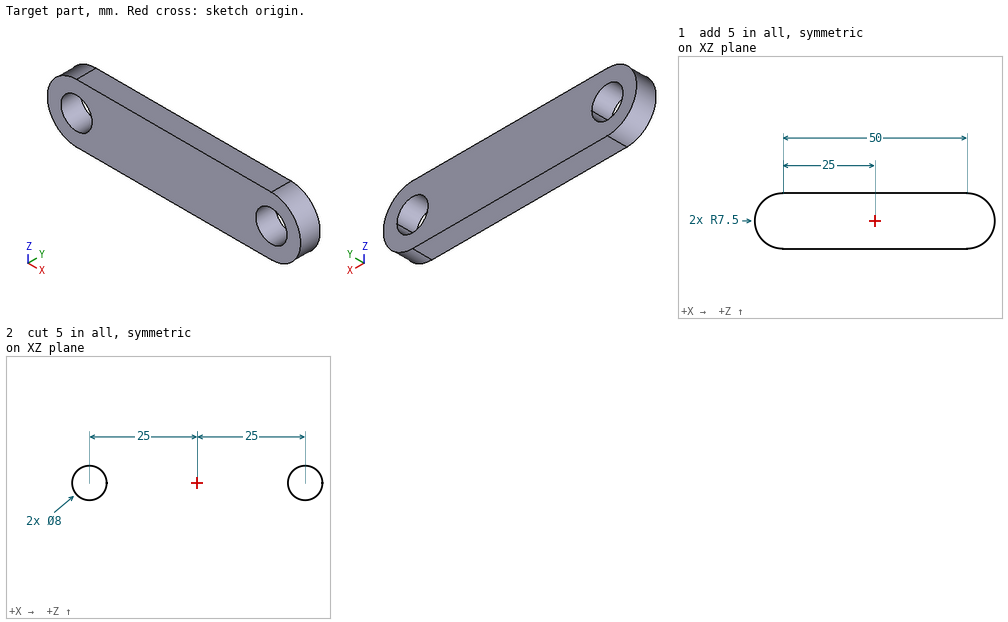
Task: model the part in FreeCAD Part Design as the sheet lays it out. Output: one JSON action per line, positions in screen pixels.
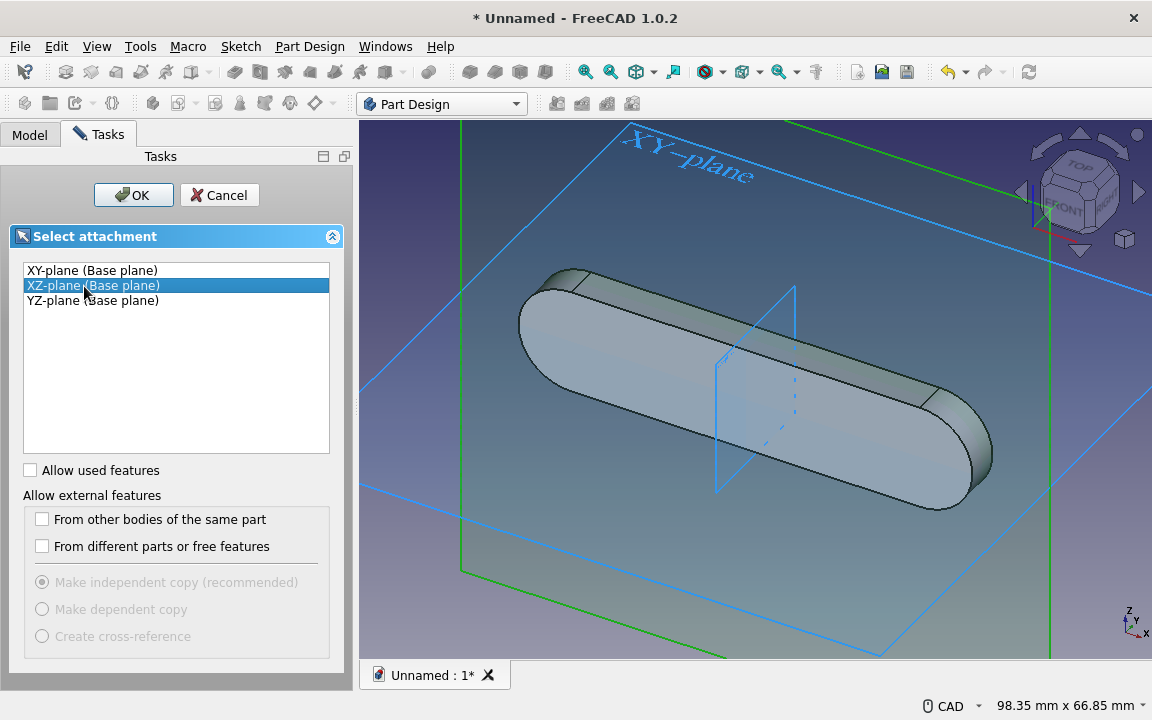
{"action": "left_click", "coordinate": [134, 195]}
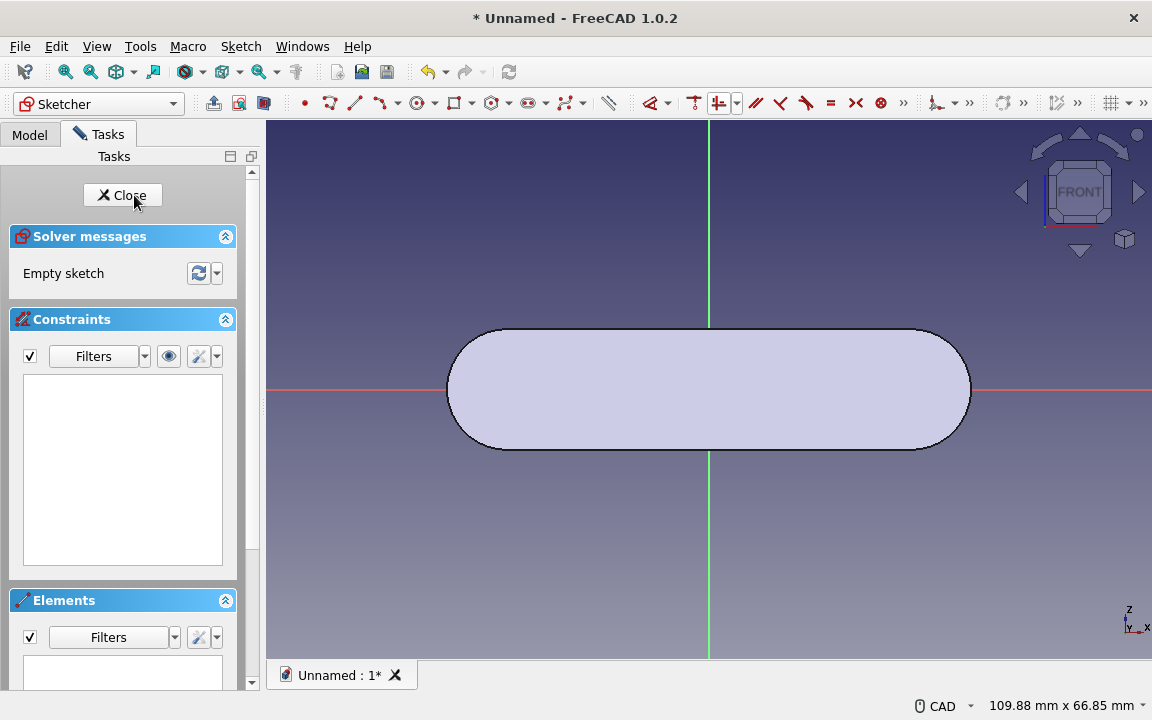
{"action": "left_click", "coordinate": [264, 104]}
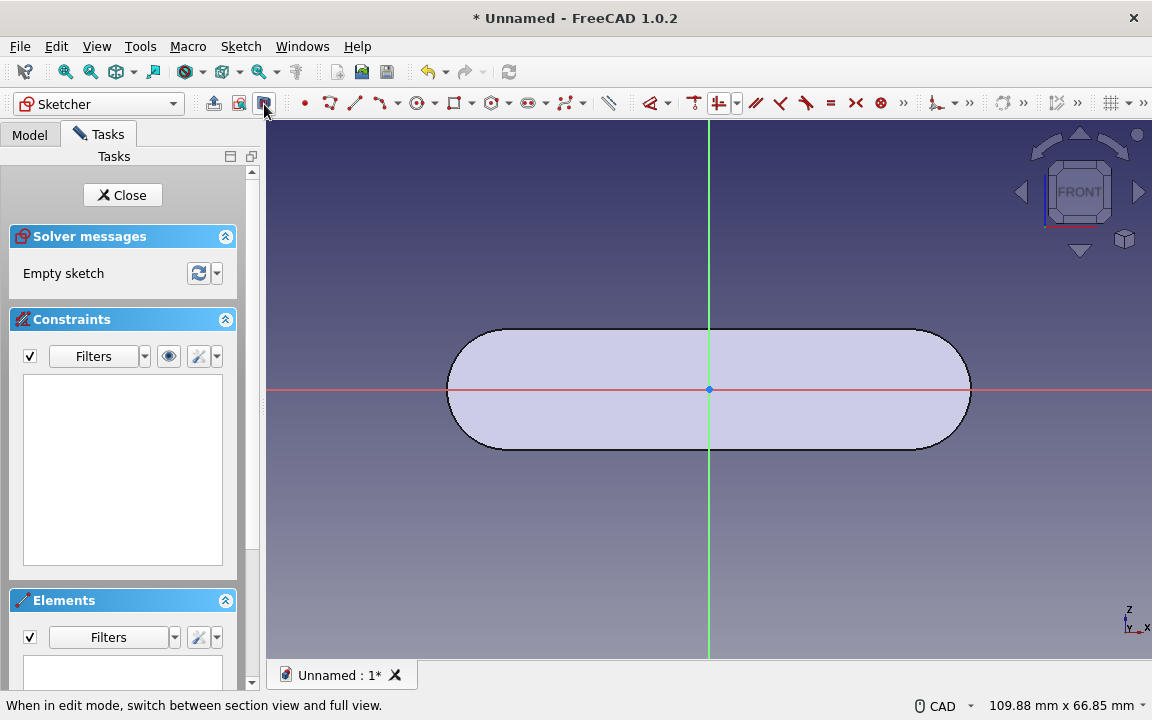
{"action": "left_click", "coordinate": [416, 104]}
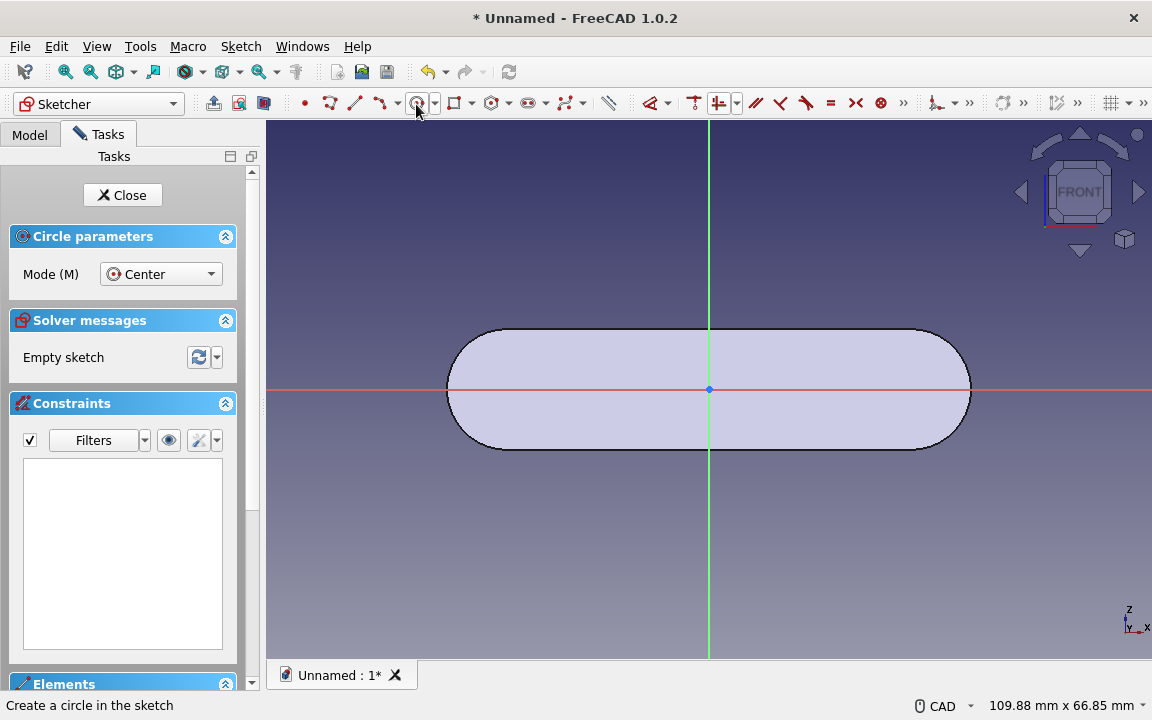
{"action": "left_click", "coordinate": [507, 390]}
{"action": "left_click", "coordinate": [530, 367]}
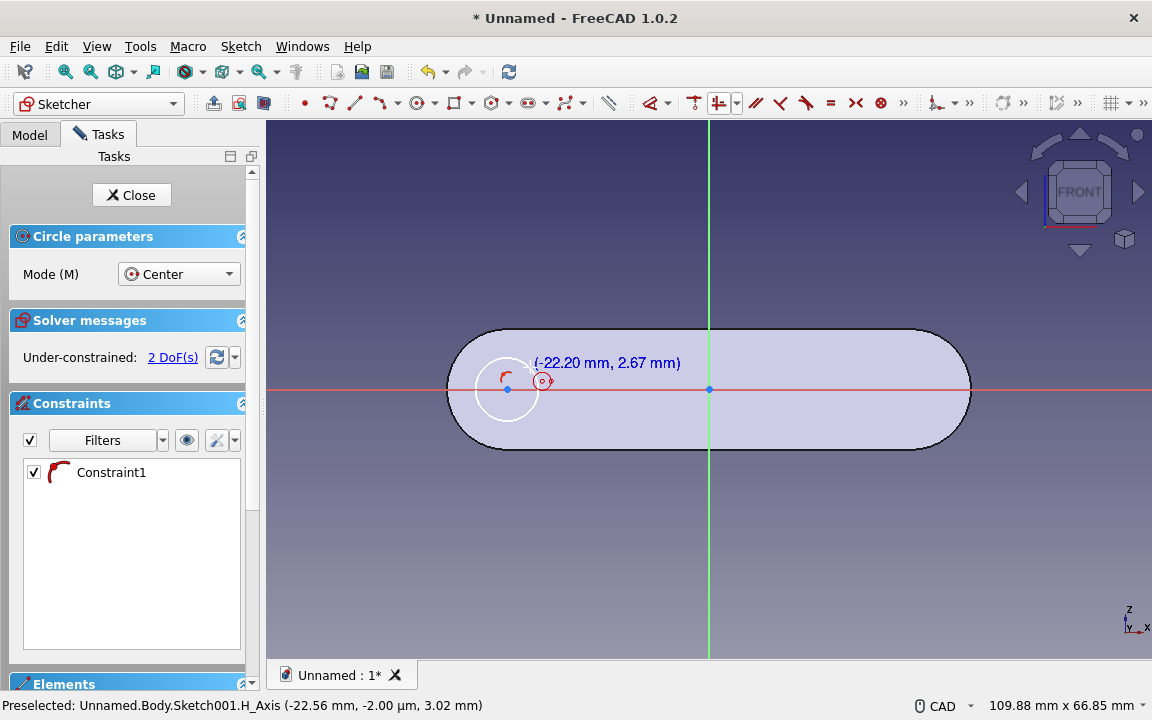
{"action": "left_click", "coordinate": [911, 390]}
{"action": "left_click", "coordinate": [933, 367]}
{"action": "key", "text": "Escape"}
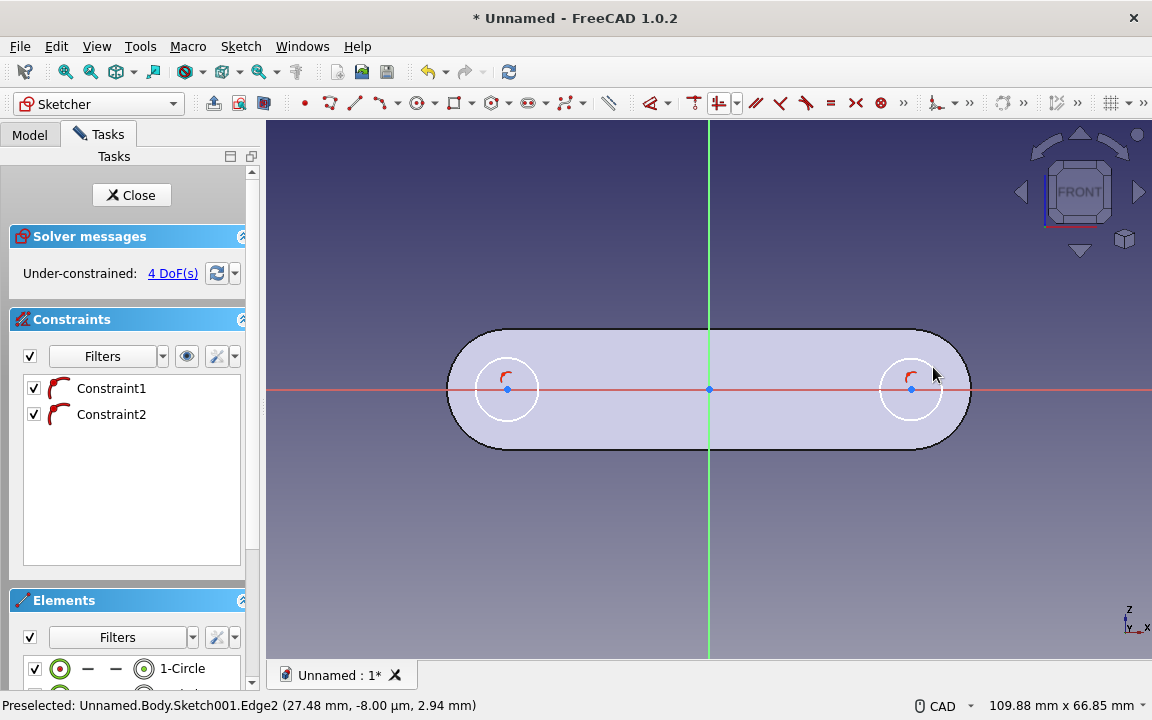
{"action": "left_click", "coordinate": [529, 367]}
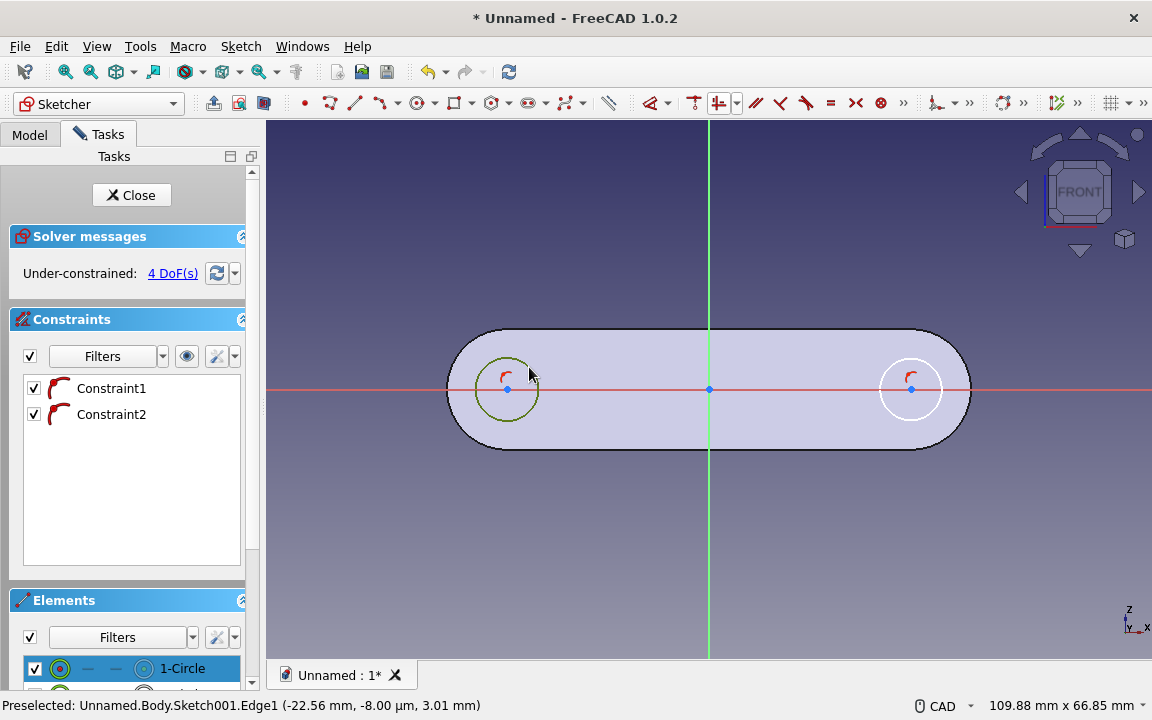
{"action": "left_click", "coordinate": [933, 368]}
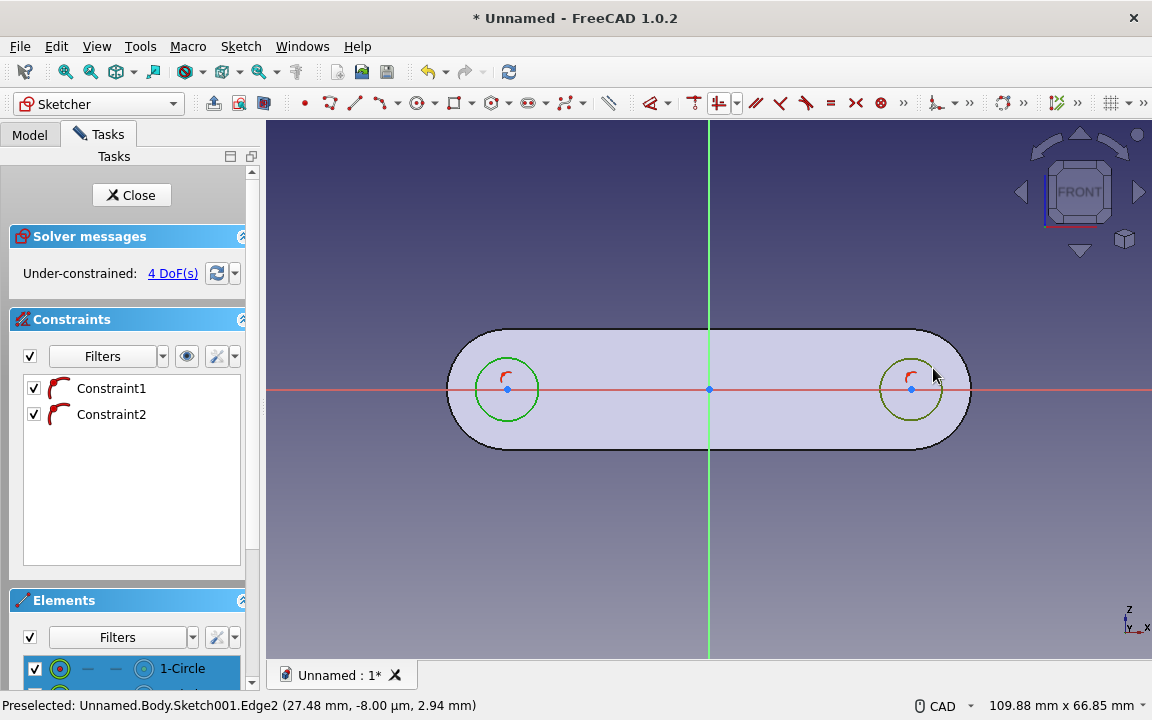
{"action": "left_click", "coordinate": [831, 104]}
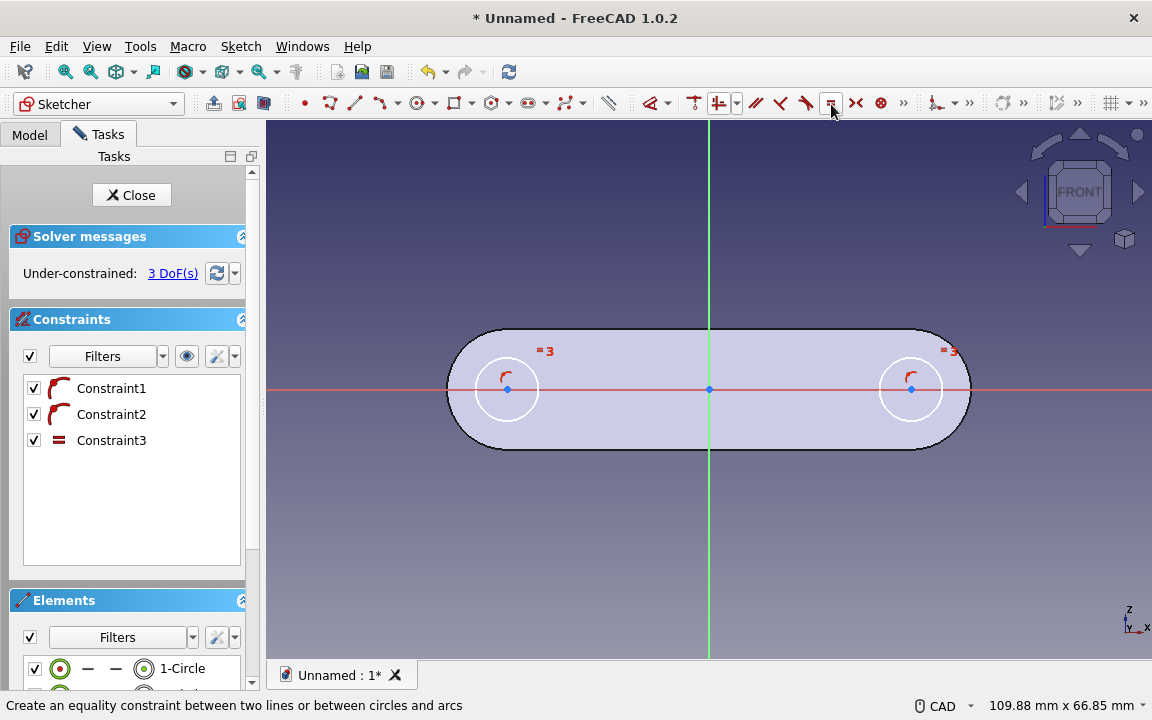
{"action": "key", "text": "d"}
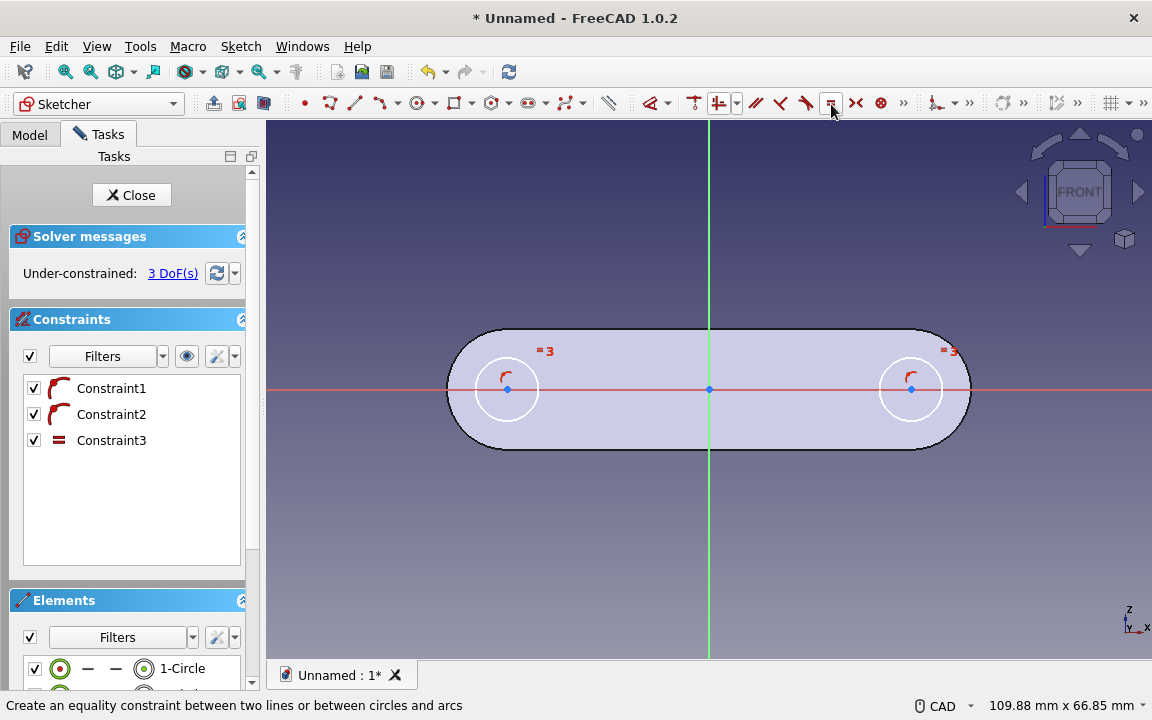
{"action": "left_click", "coordinate": [529, 367]}
{"action": "left_click", "coordinate": [551, 344]}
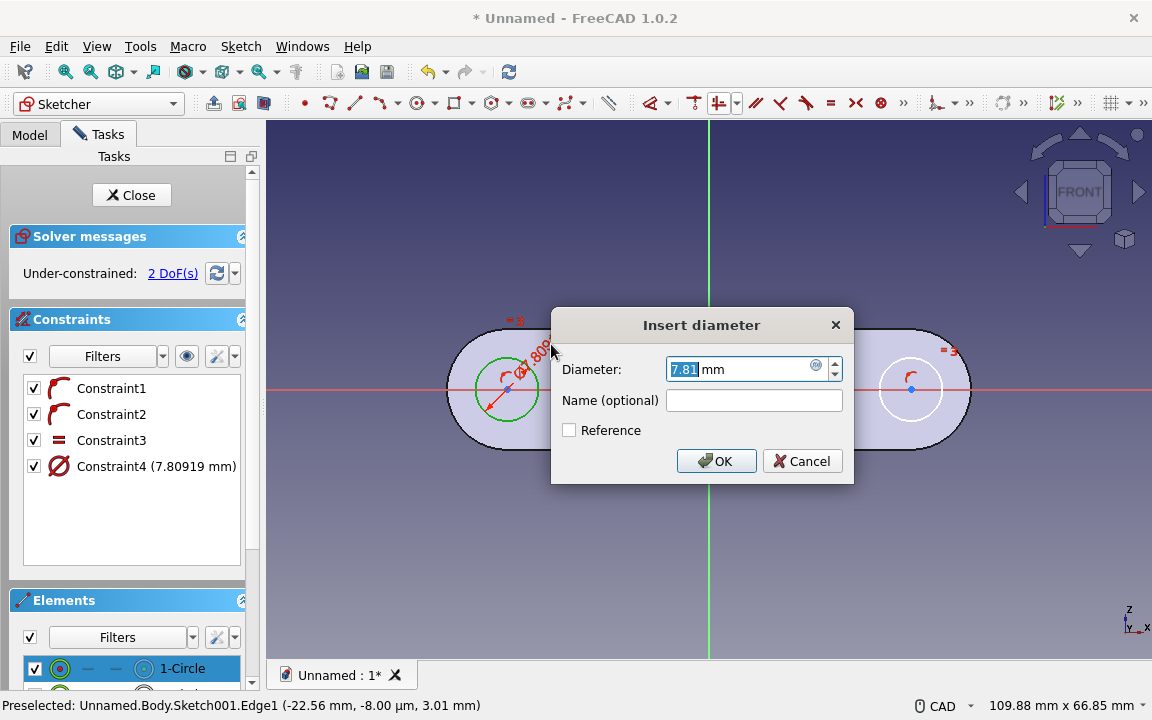
{"action": "type", "text": "8"}
{"action": "key", "text": "Return"}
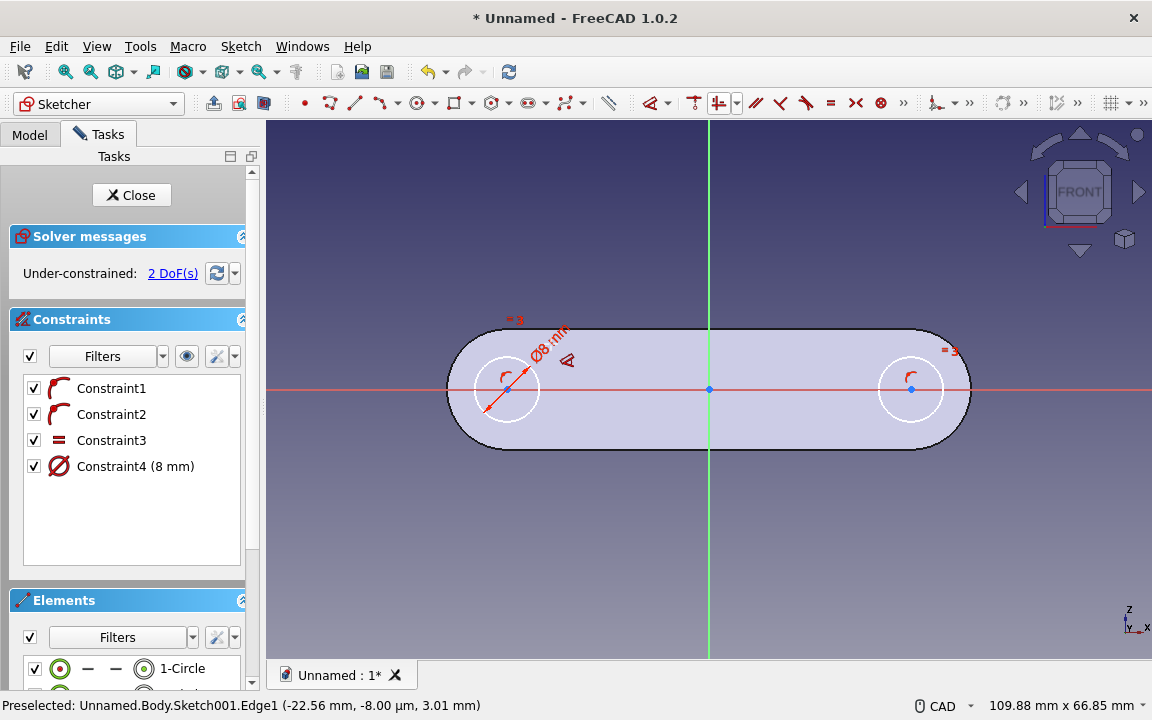
{"action": "left_click", "coordinate": [507, 390]}
{"action": "left_click", "coordinate": [608, 424]}